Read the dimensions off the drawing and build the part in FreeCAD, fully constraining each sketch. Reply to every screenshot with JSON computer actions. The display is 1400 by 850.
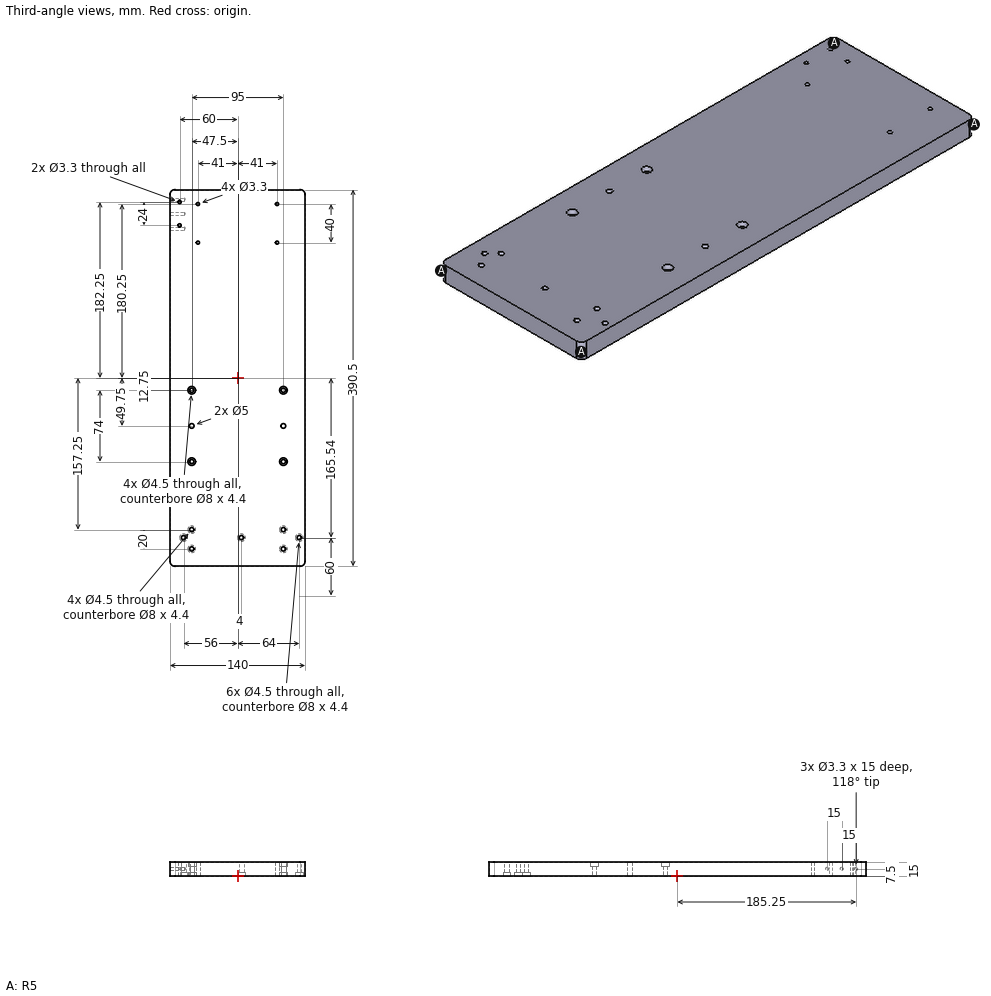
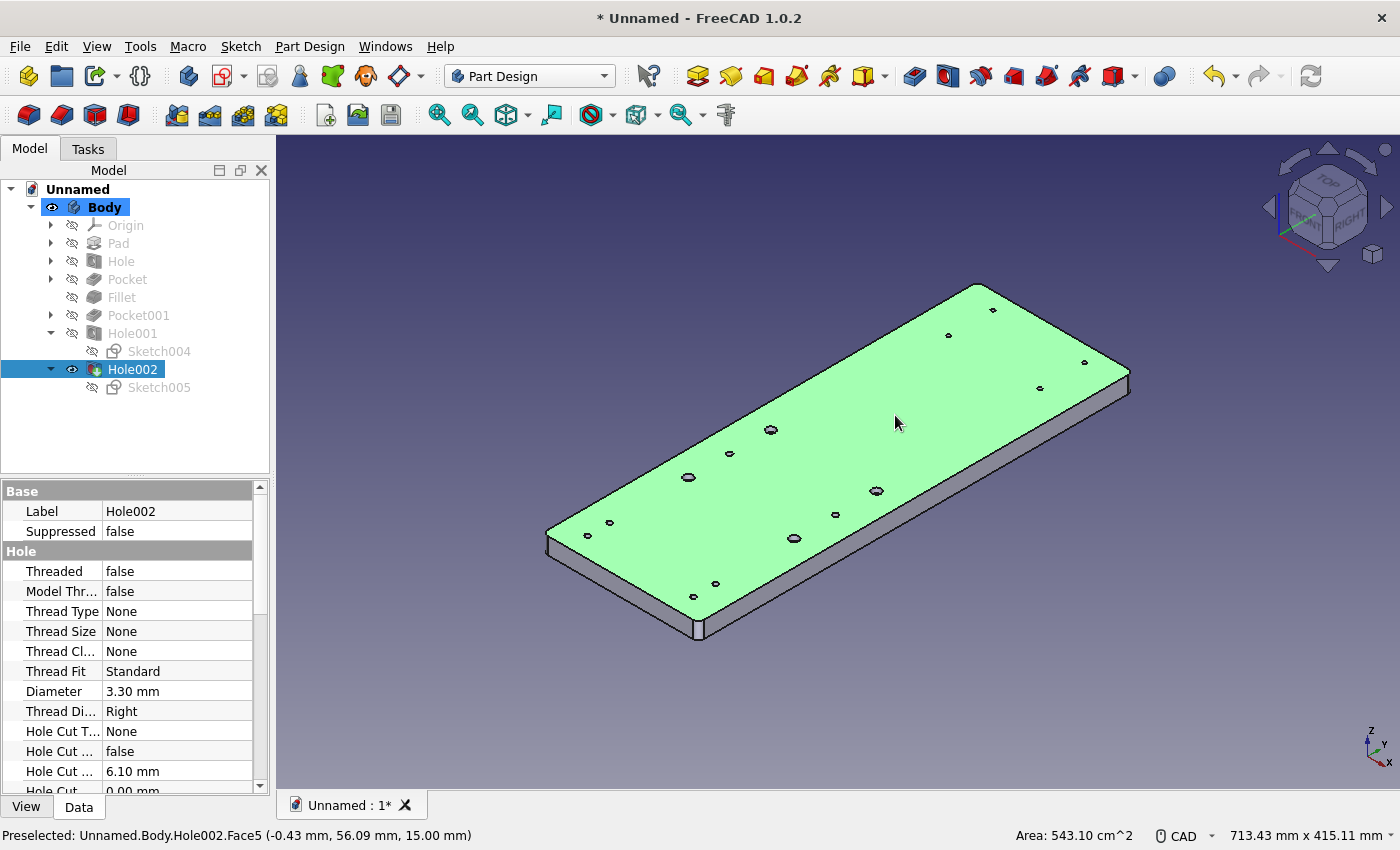
{"action": "left_click", "coordinate": [222, 76]}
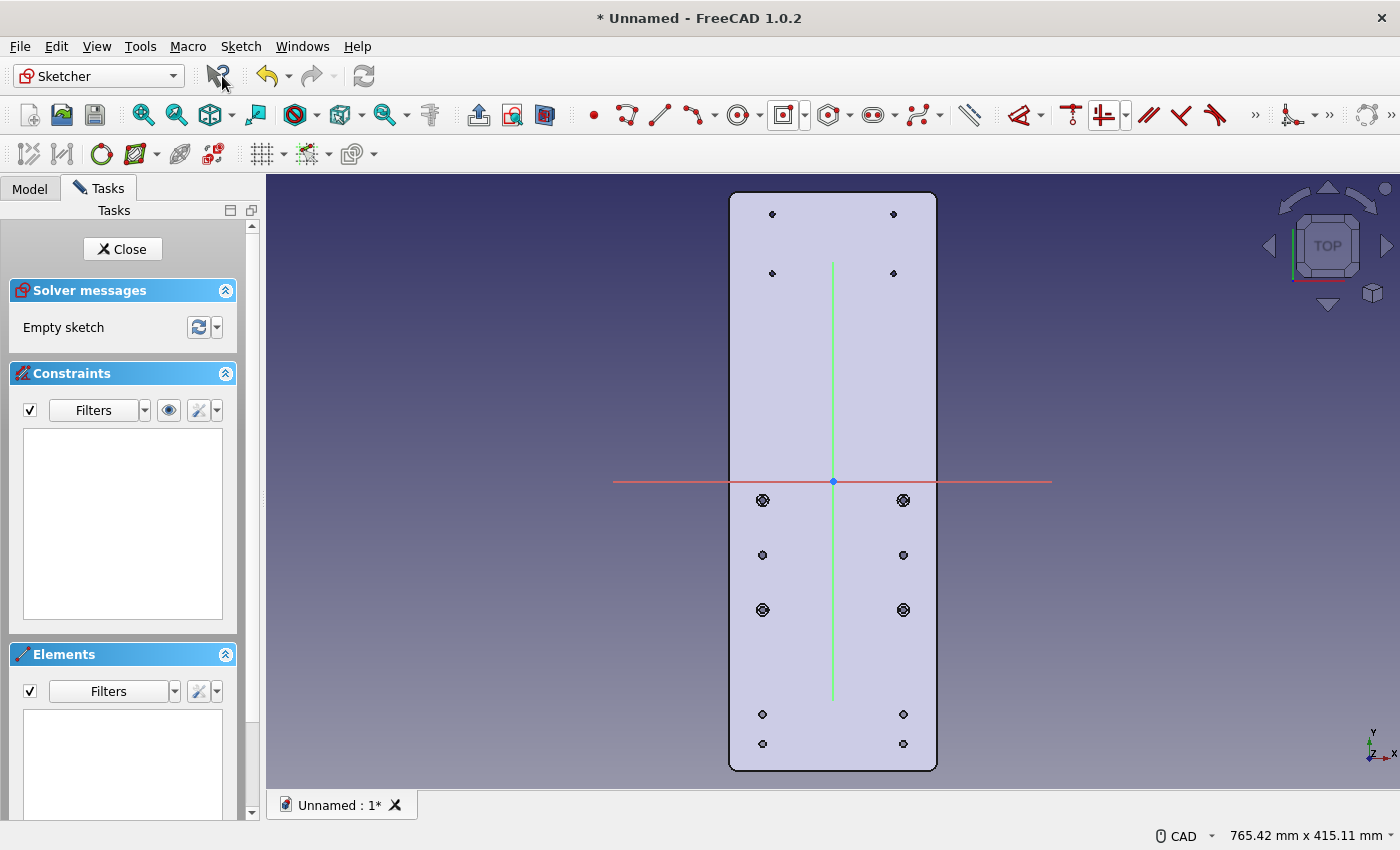
{"action": "scroll", "coordinate": [742, 202], "scroll_direction": "up", "scroll_amount": 11}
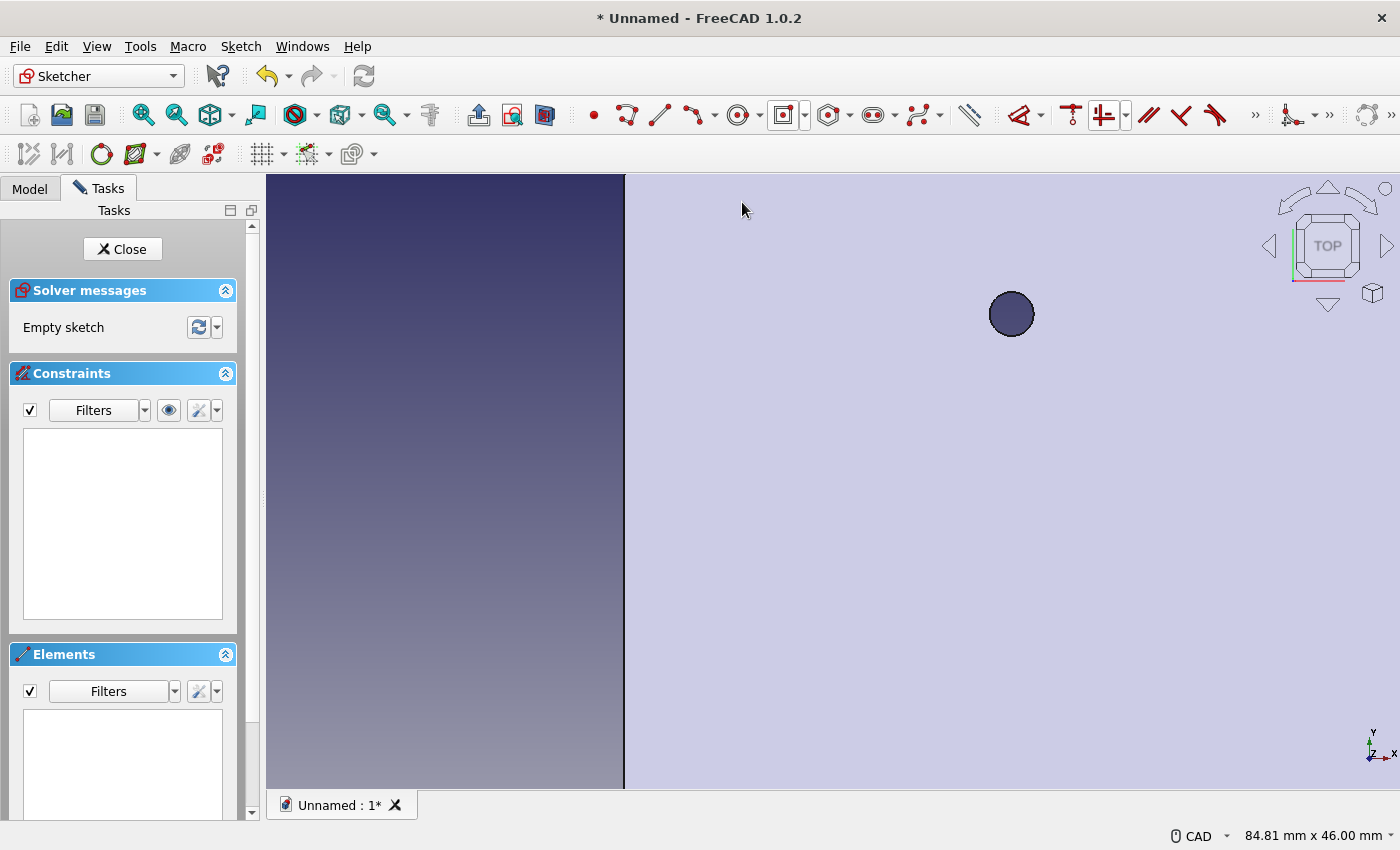
{"action": "left_click", "coordinate": [738, 116]}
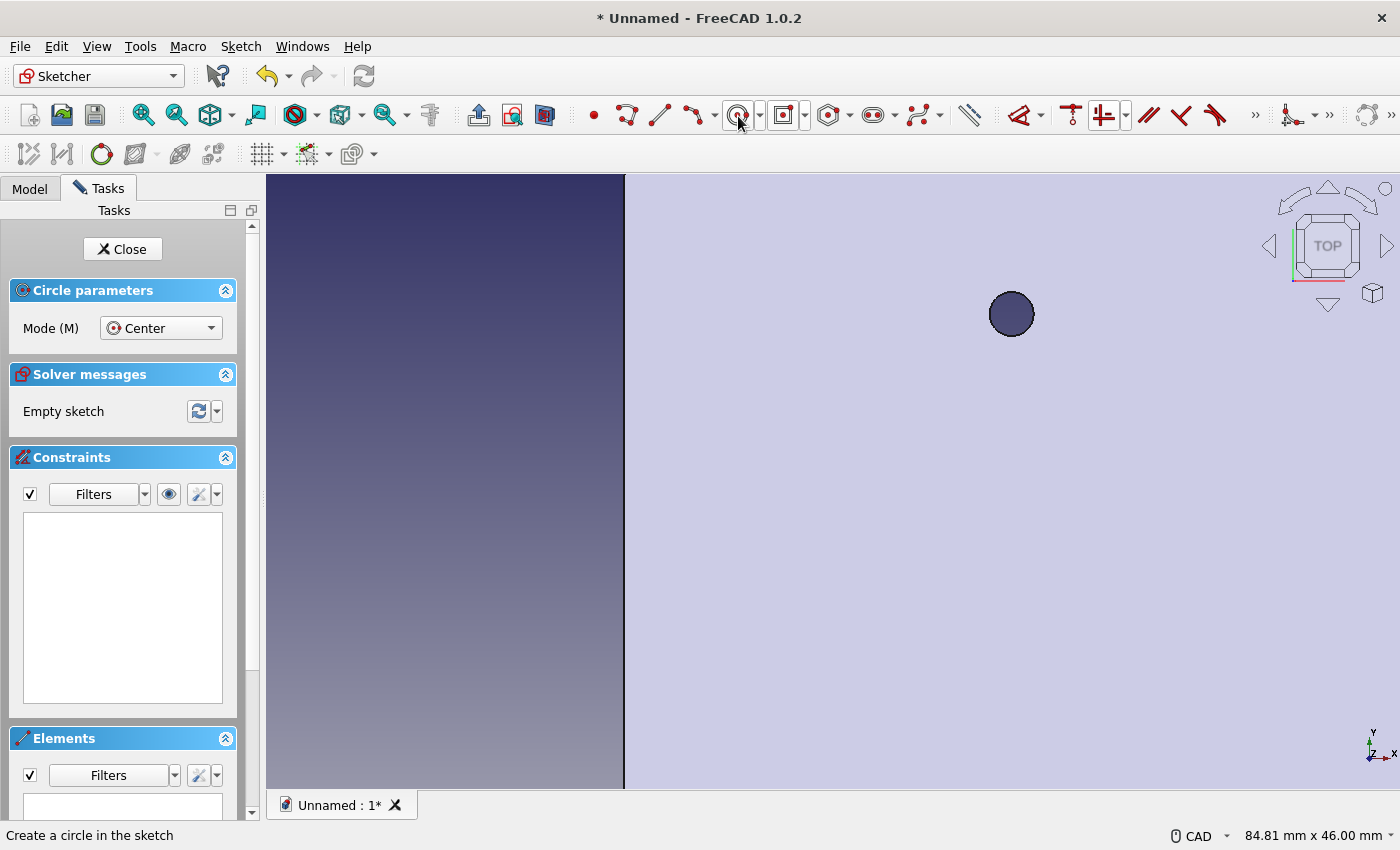
{"action": "left_click", "coordinate": [758, 287]}
{"action": "mouse_move", "coordinate": [773, 272]}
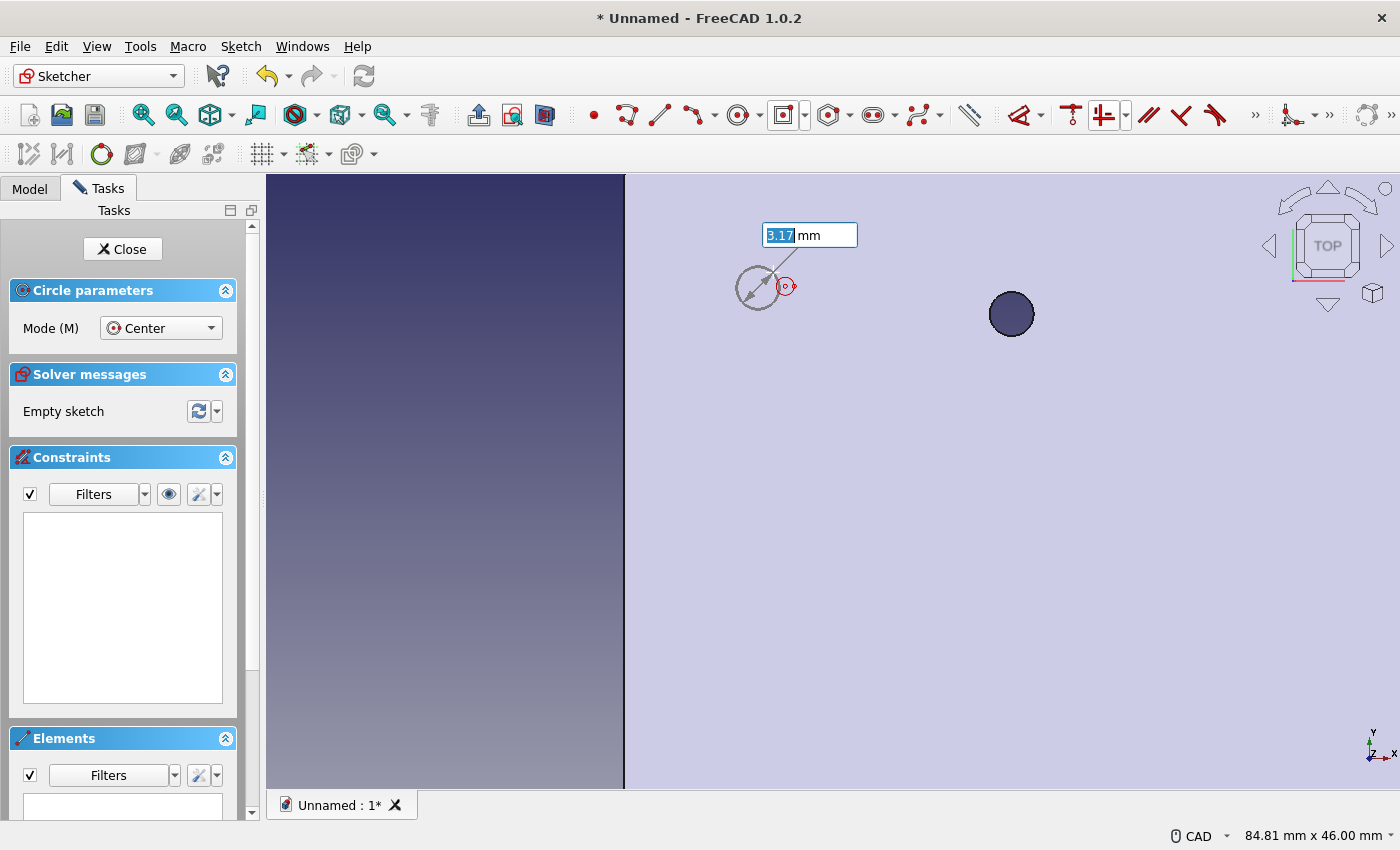
{"action": "type", "text": "3.3"}
{"action": "key", "text": "Return"}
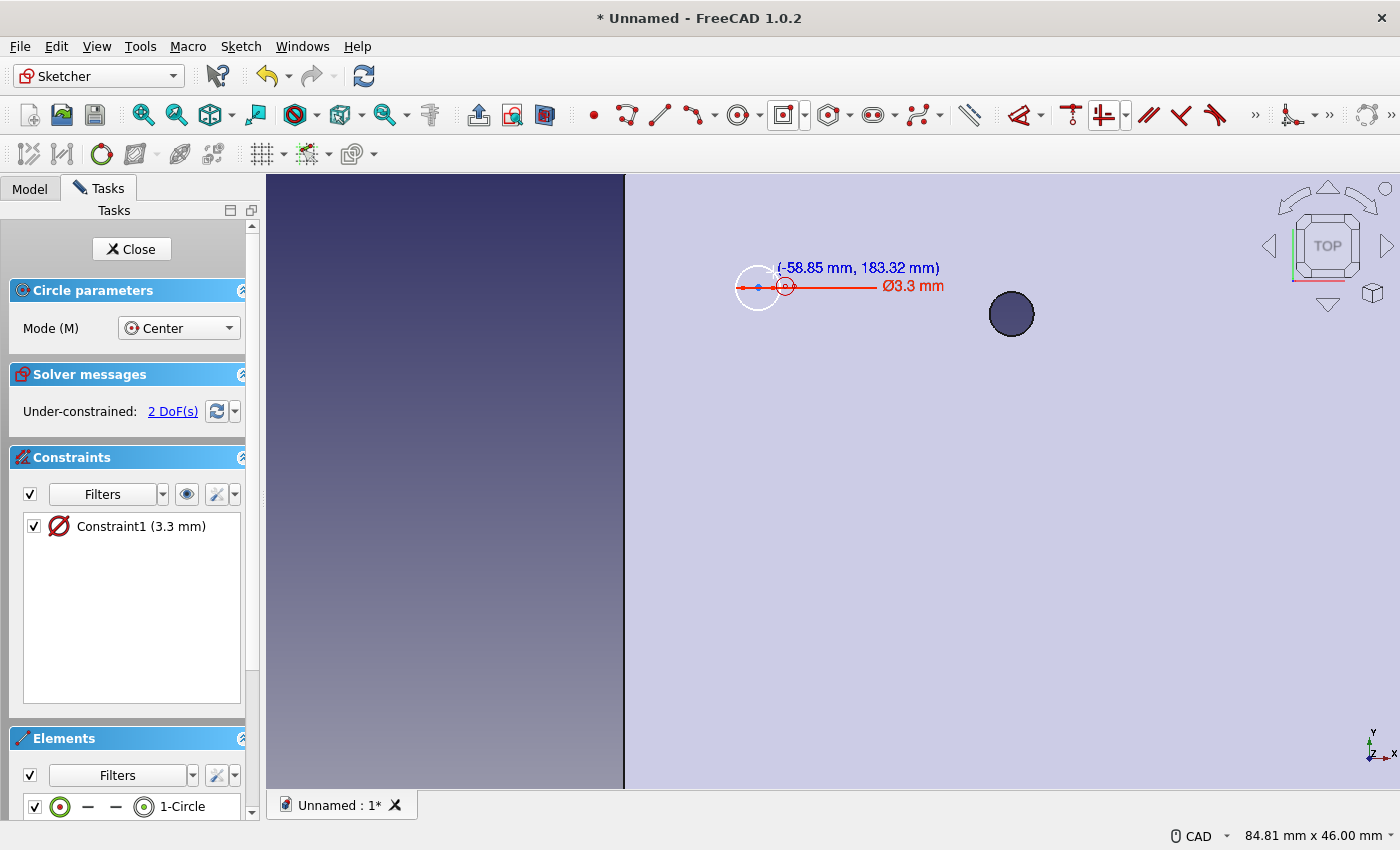
{"action": "left_click", "coordinate": [758, 608]}
{"action": "mouse_move", "coordinate": [773, 593]}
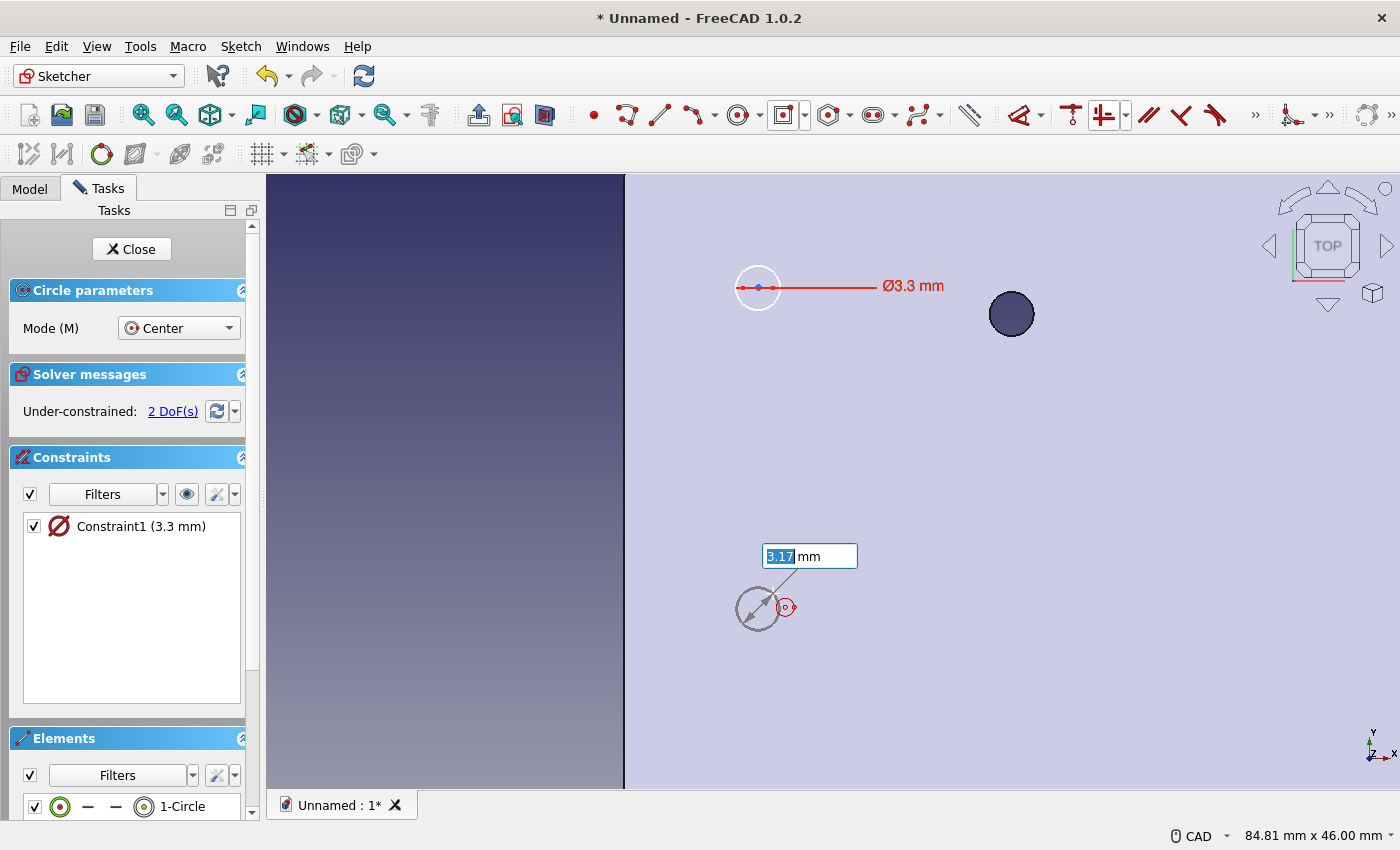
{"action": "type", "text": "3.3"}
{"action": "key", "text": "Return"}
{"action": "key", "text": "Escape"}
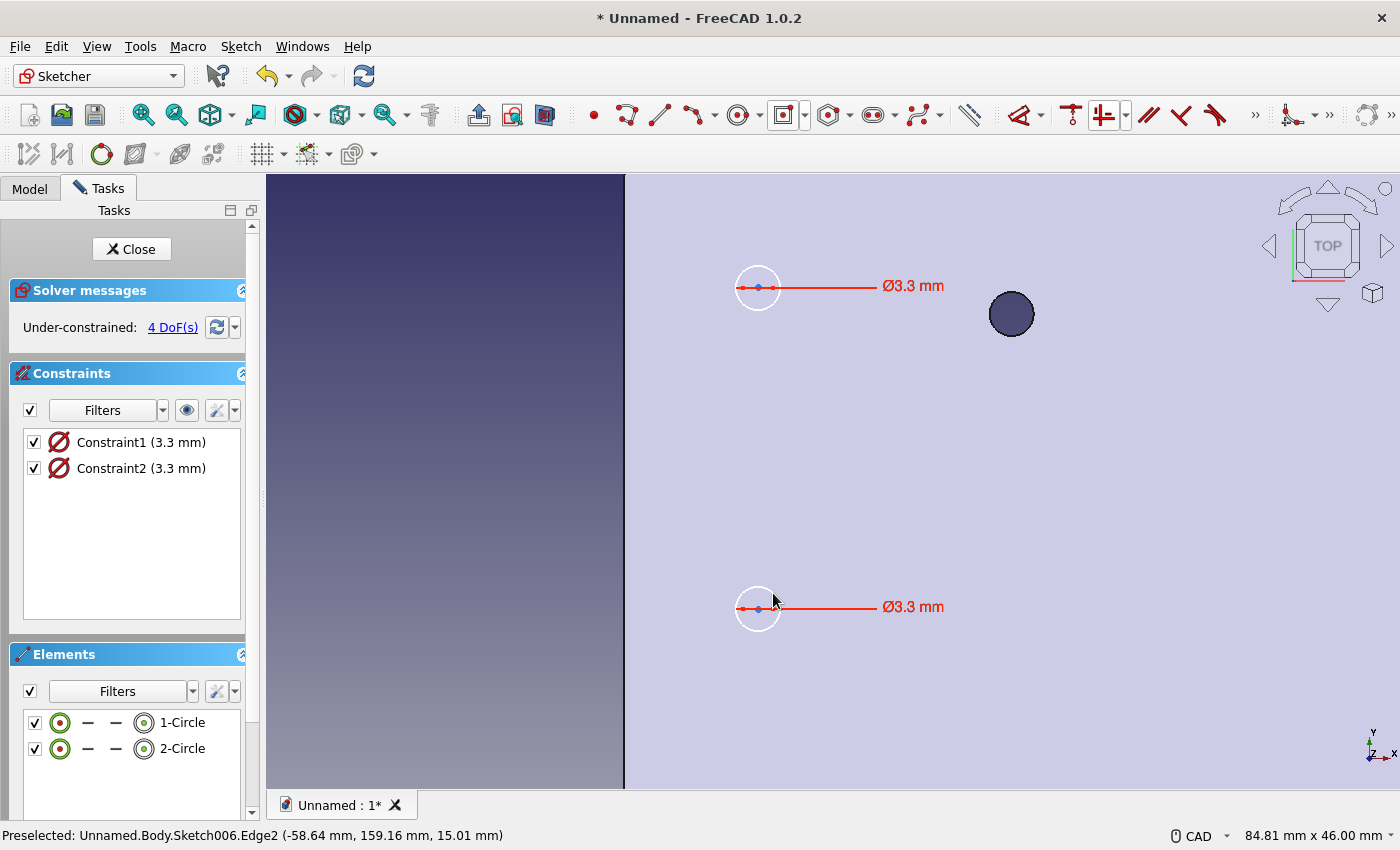
{"action": "left_click", "coordinate": [758, 288]}